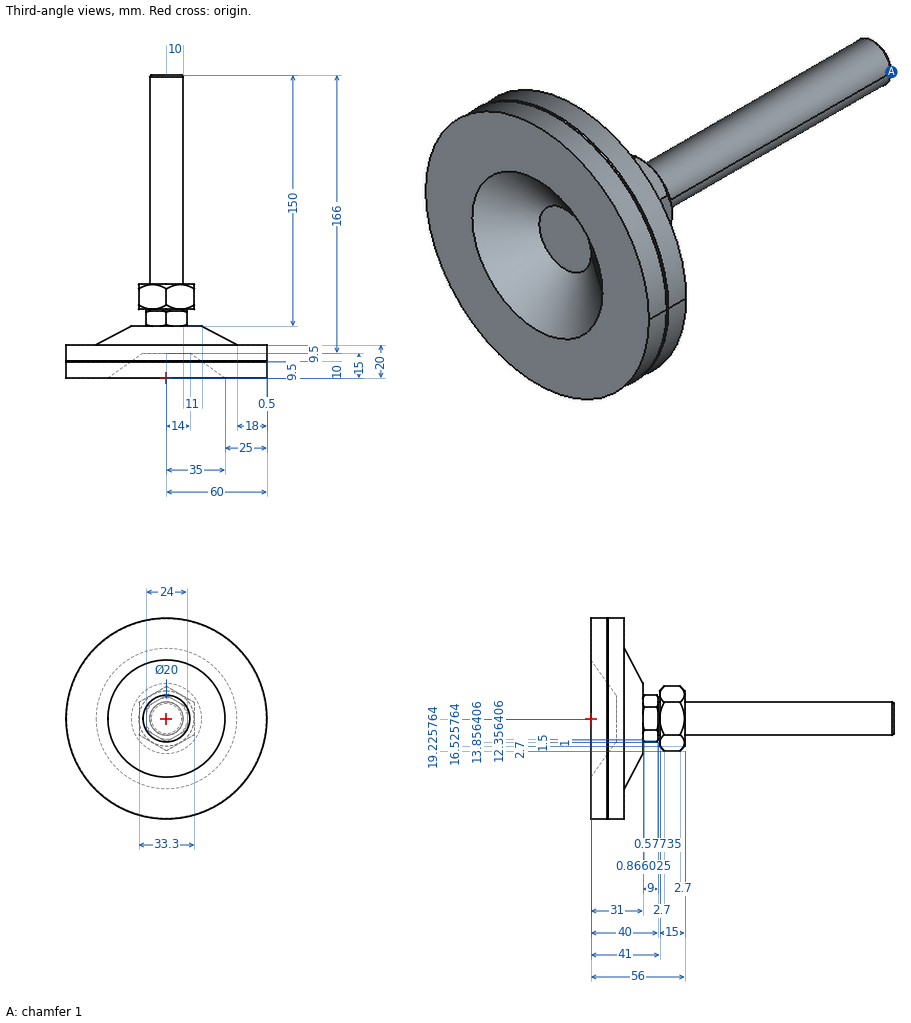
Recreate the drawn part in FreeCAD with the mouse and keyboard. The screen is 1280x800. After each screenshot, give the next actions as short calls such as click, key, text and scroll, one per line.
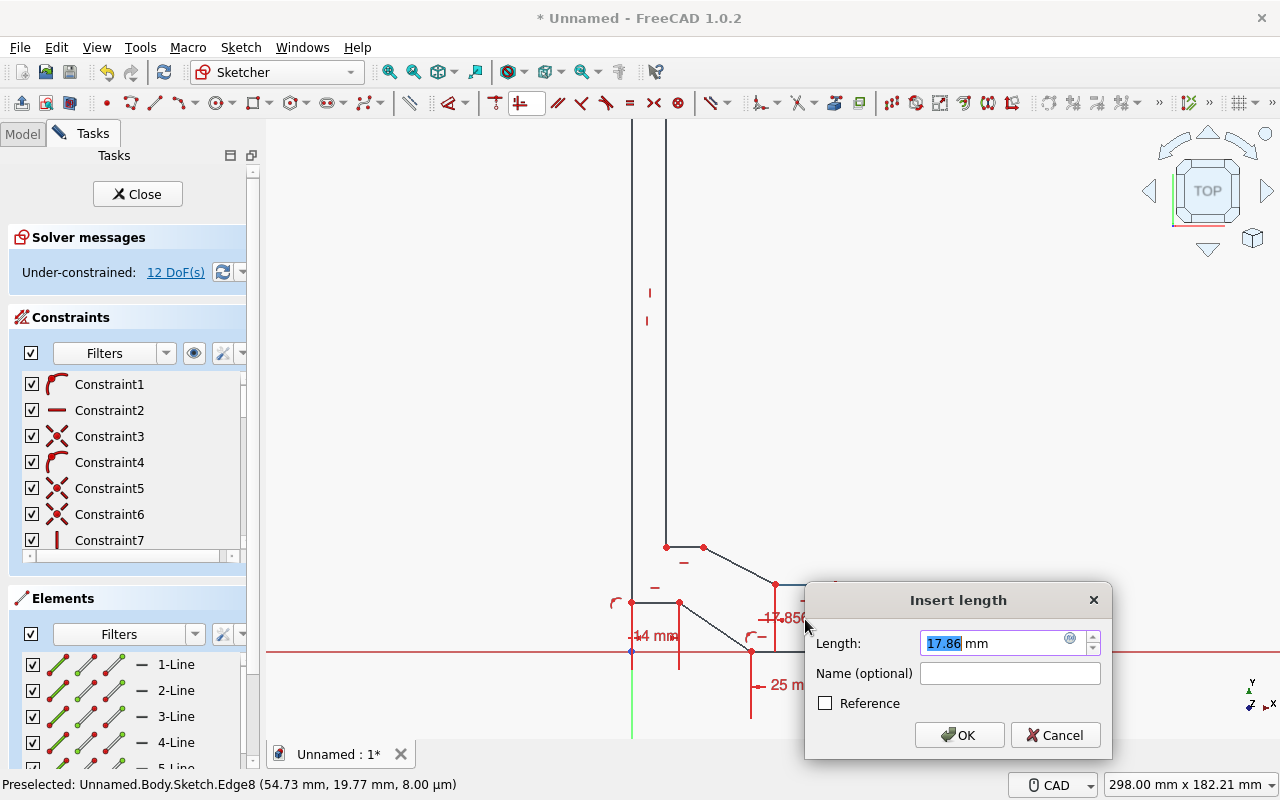
text(18)
key(Return)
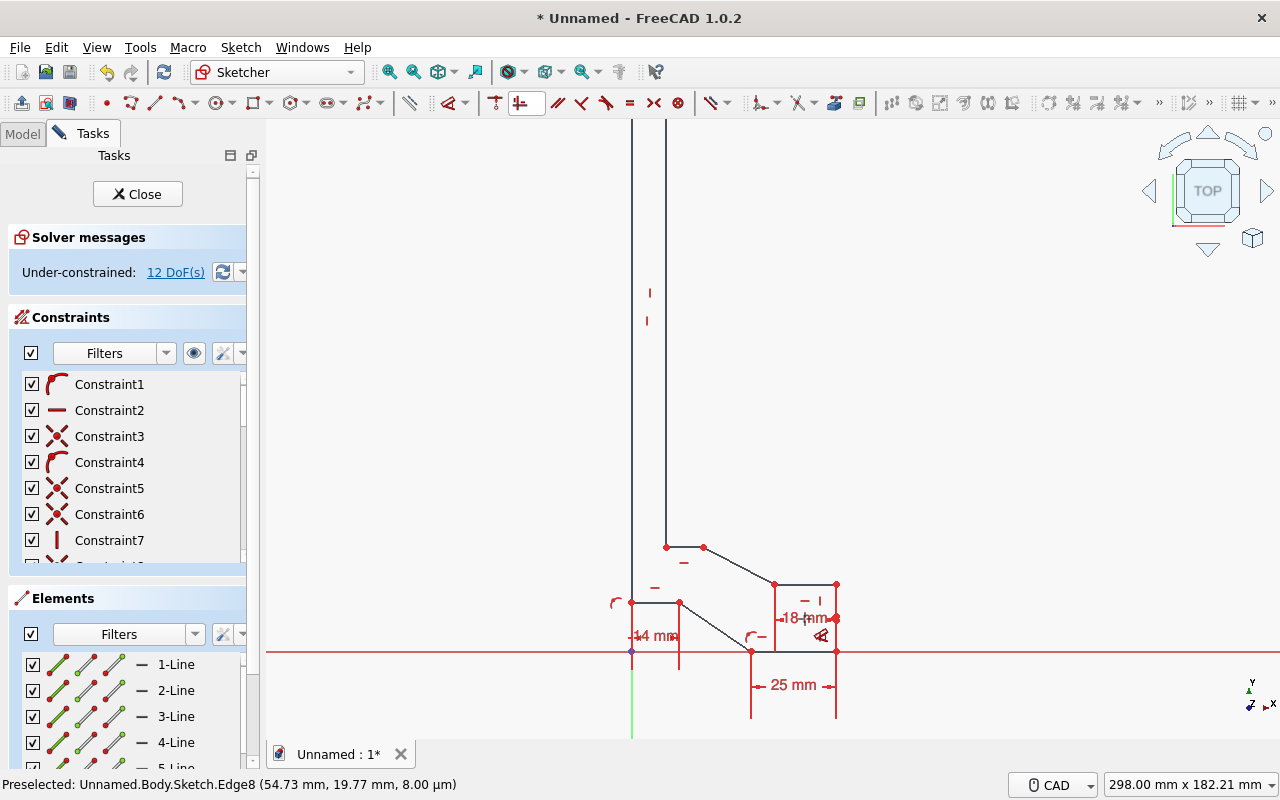
scroll(692, 547, up, 2)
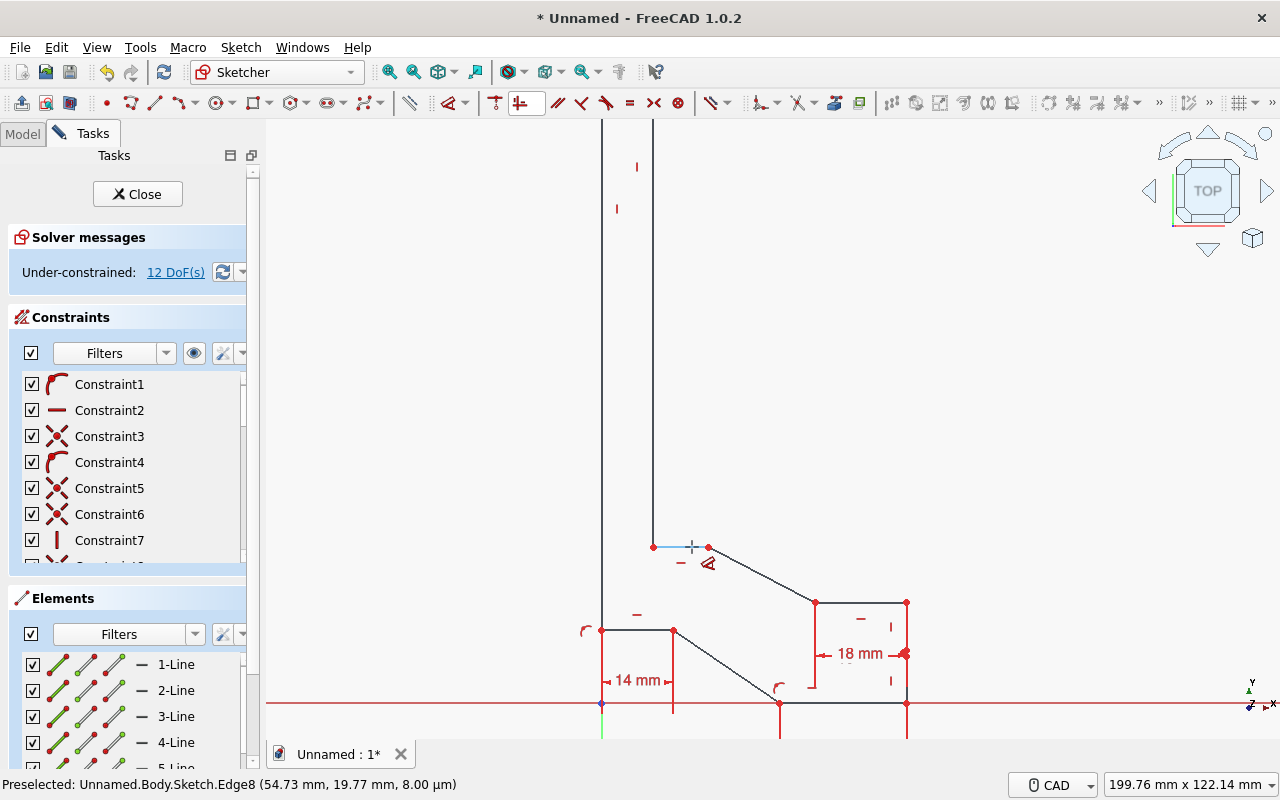
click(692, 547)
click(681, 581)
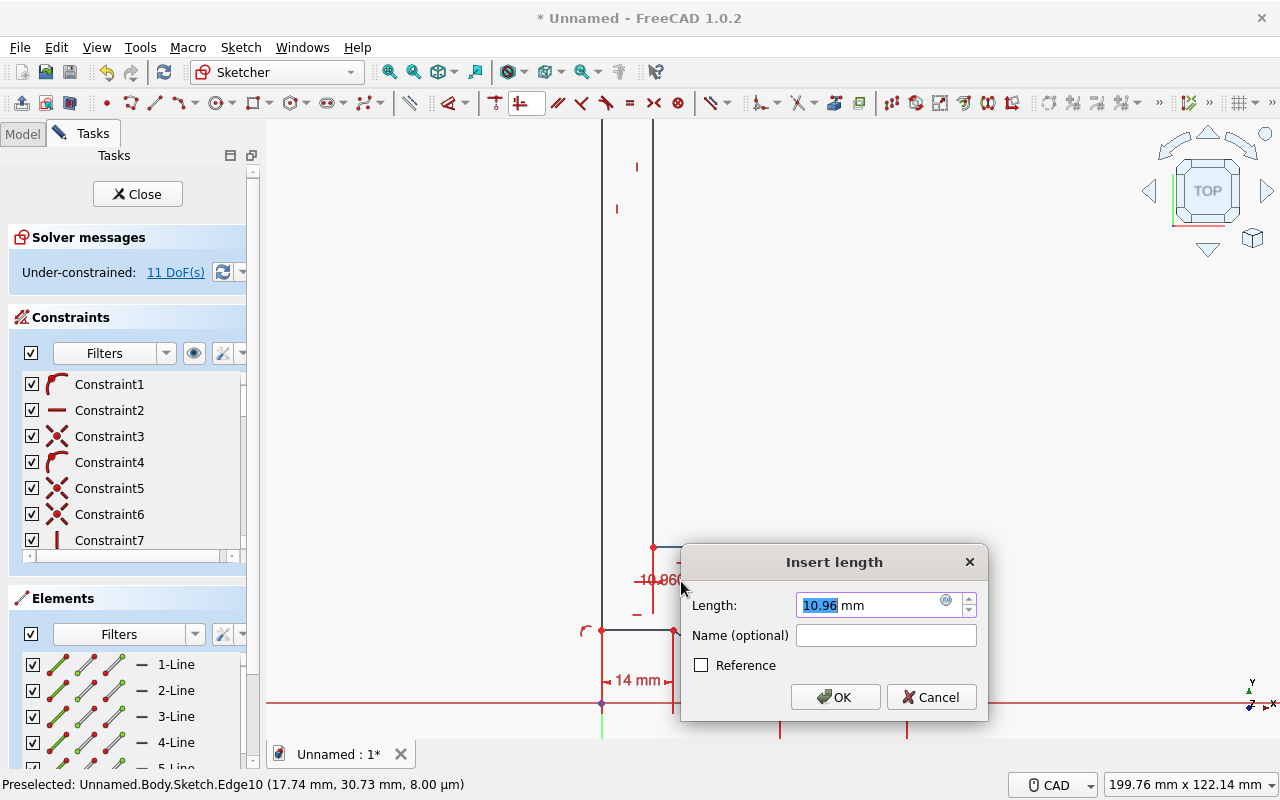
text(11)
key(Return)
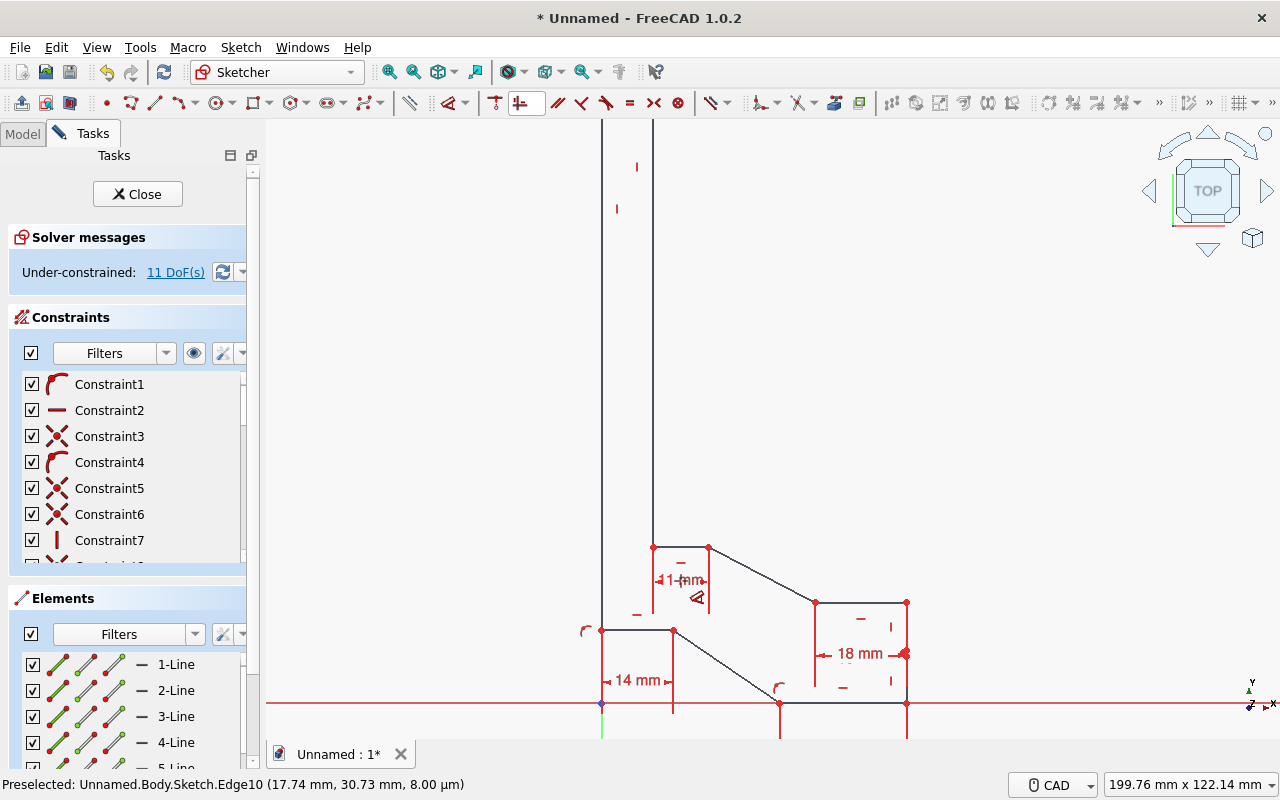
scroll(664, 580, down, 4)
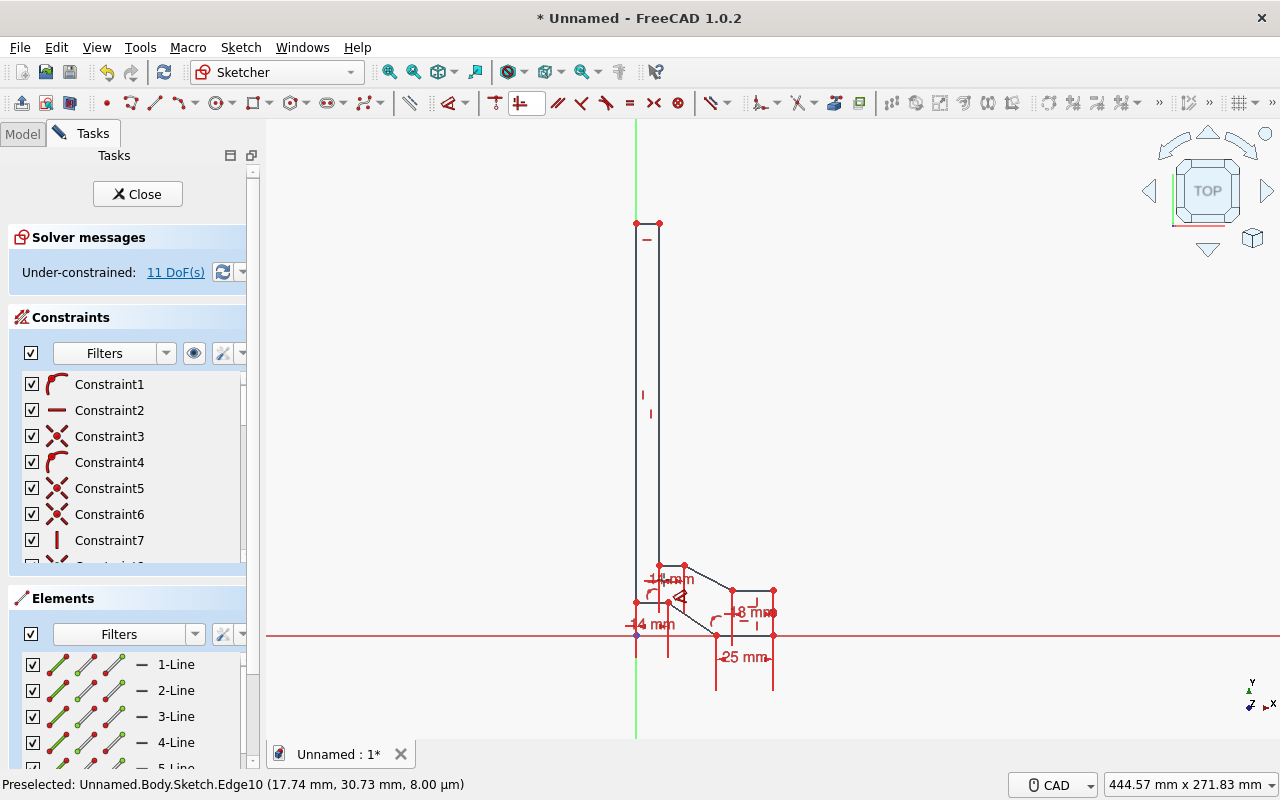
scroll(652, 224, up, 4)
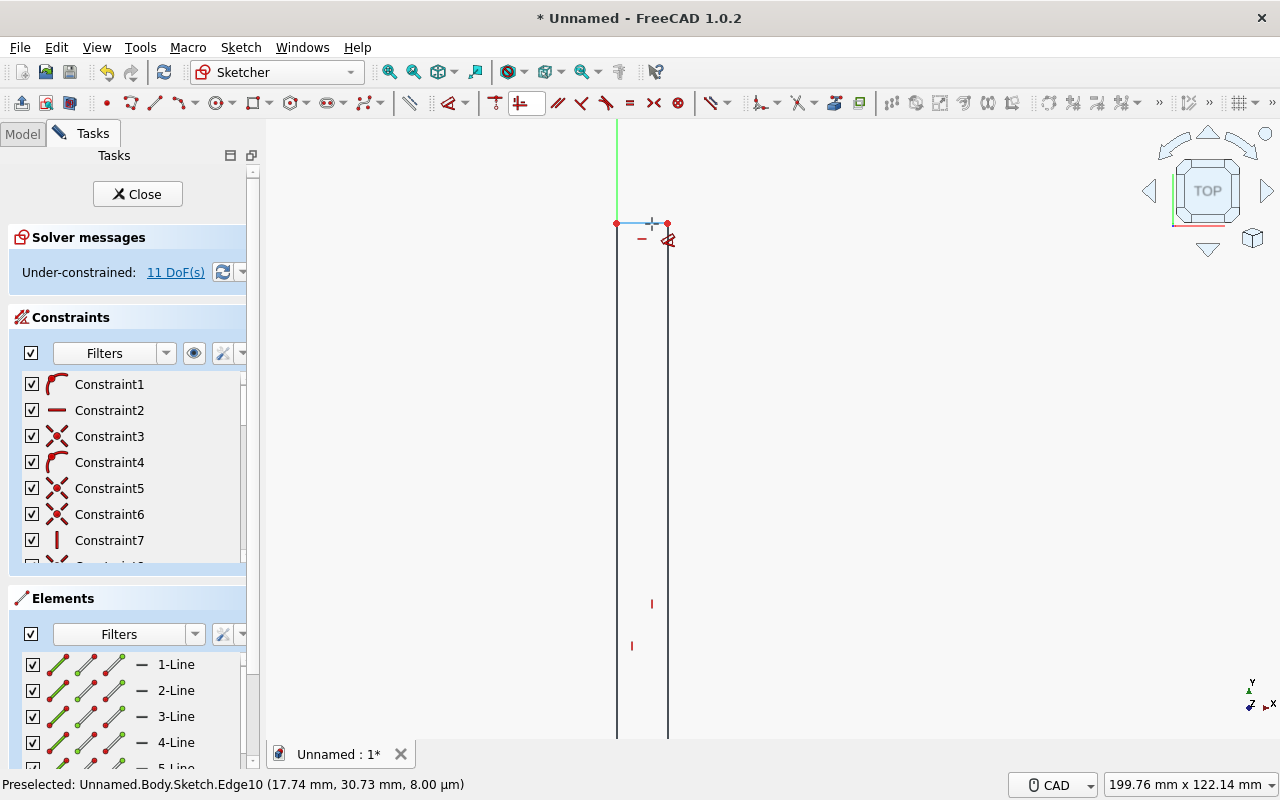
click(652, 223)
click(642, 189)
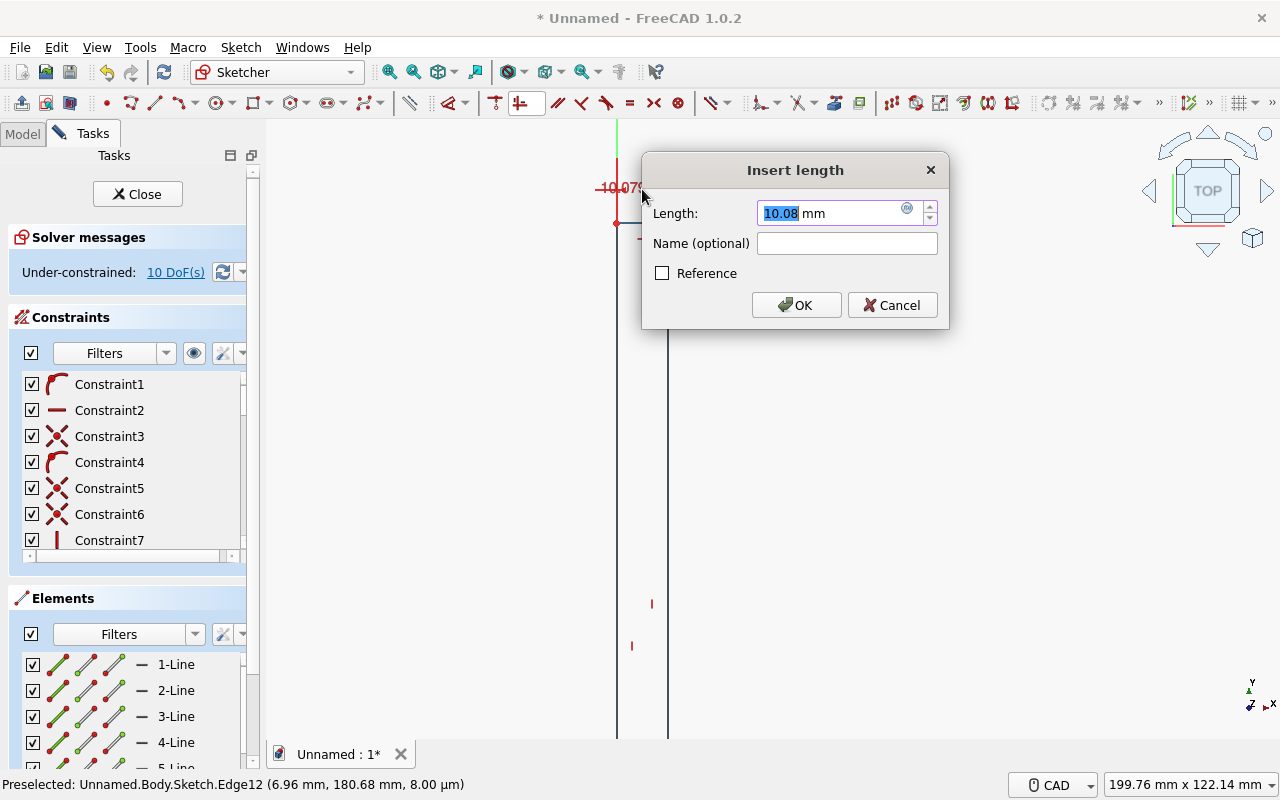
text(10)
key(Return)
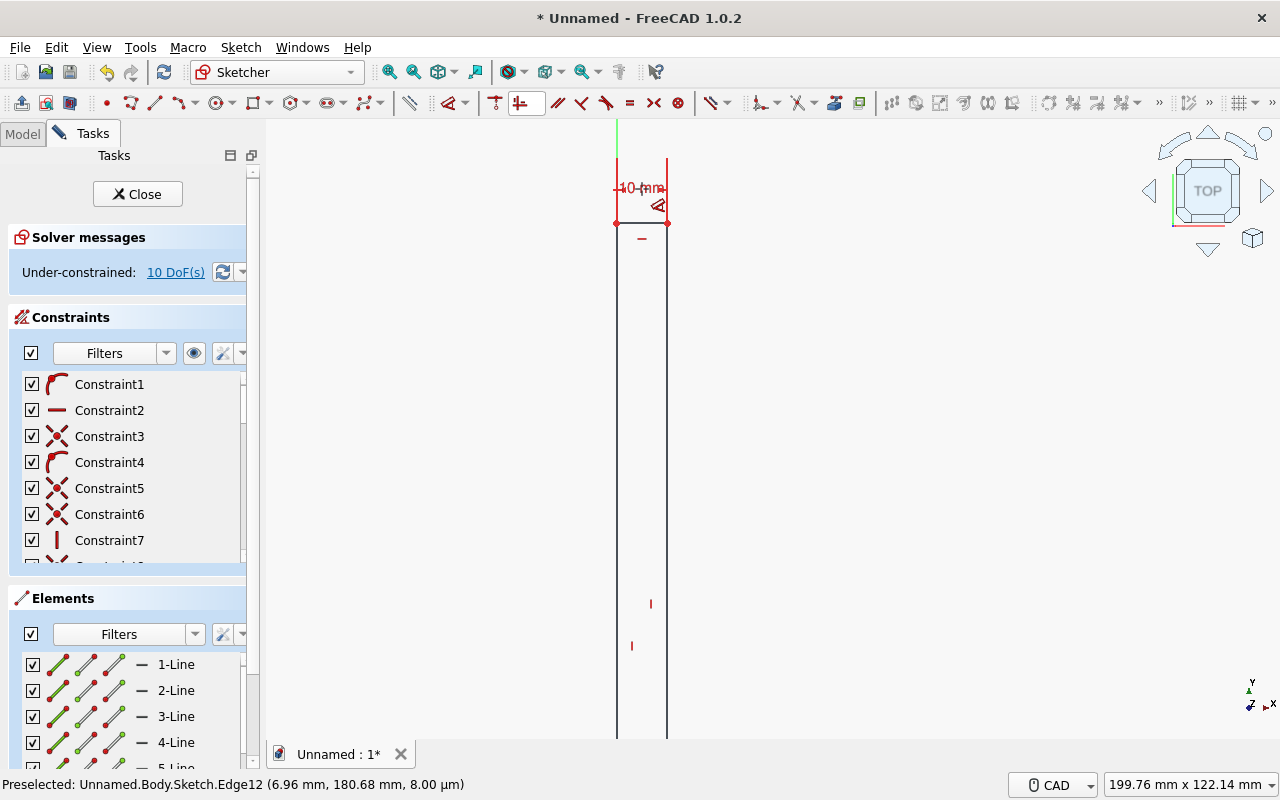
scroll(652, 223, down, 4)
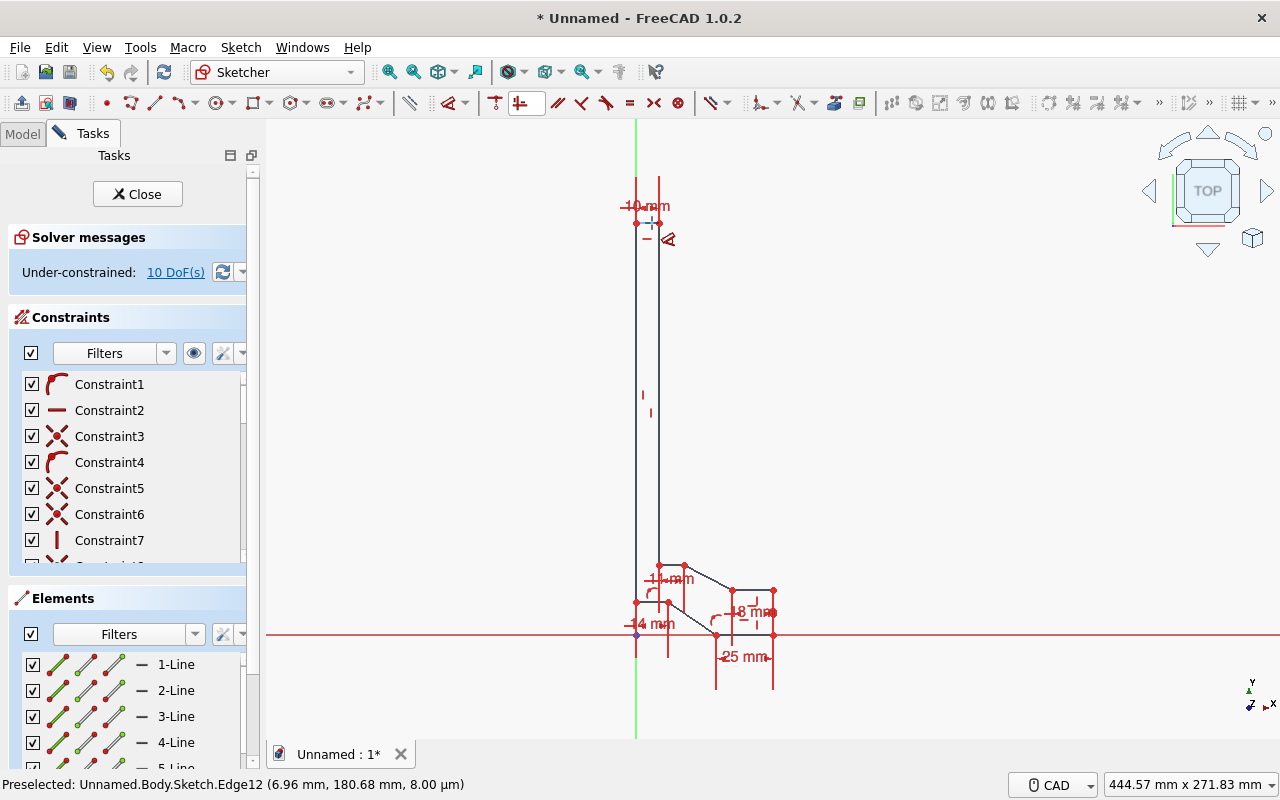
scroll(773, 629, up, 4)